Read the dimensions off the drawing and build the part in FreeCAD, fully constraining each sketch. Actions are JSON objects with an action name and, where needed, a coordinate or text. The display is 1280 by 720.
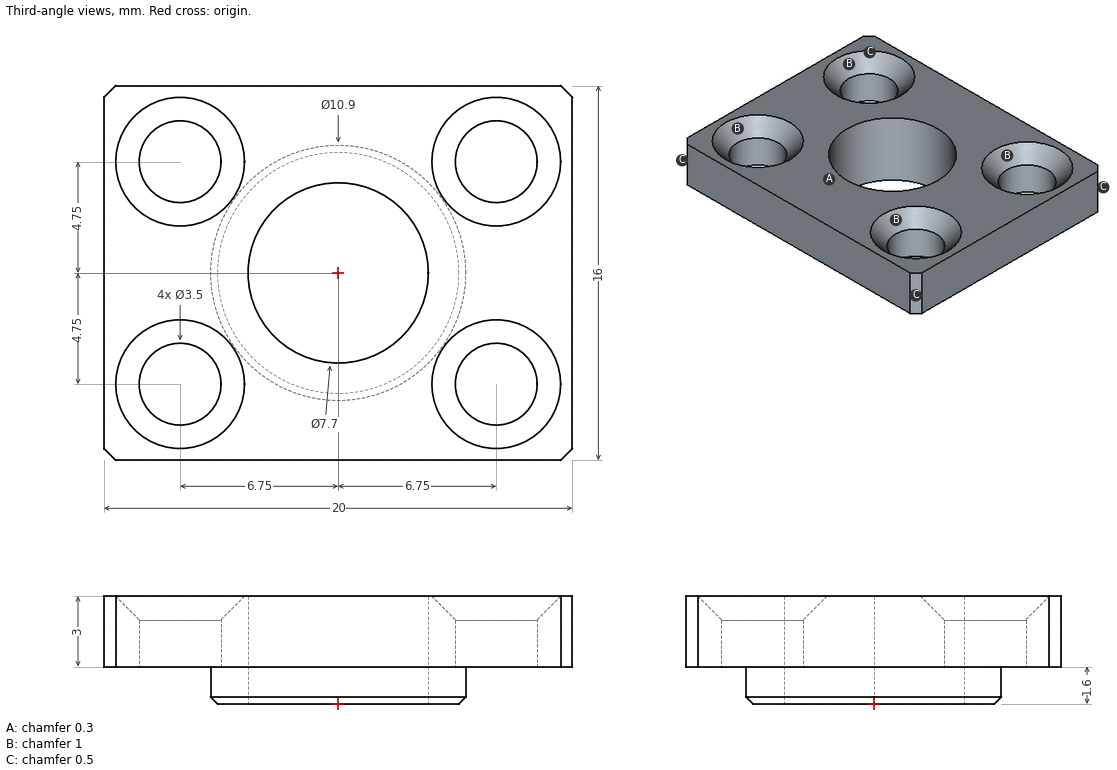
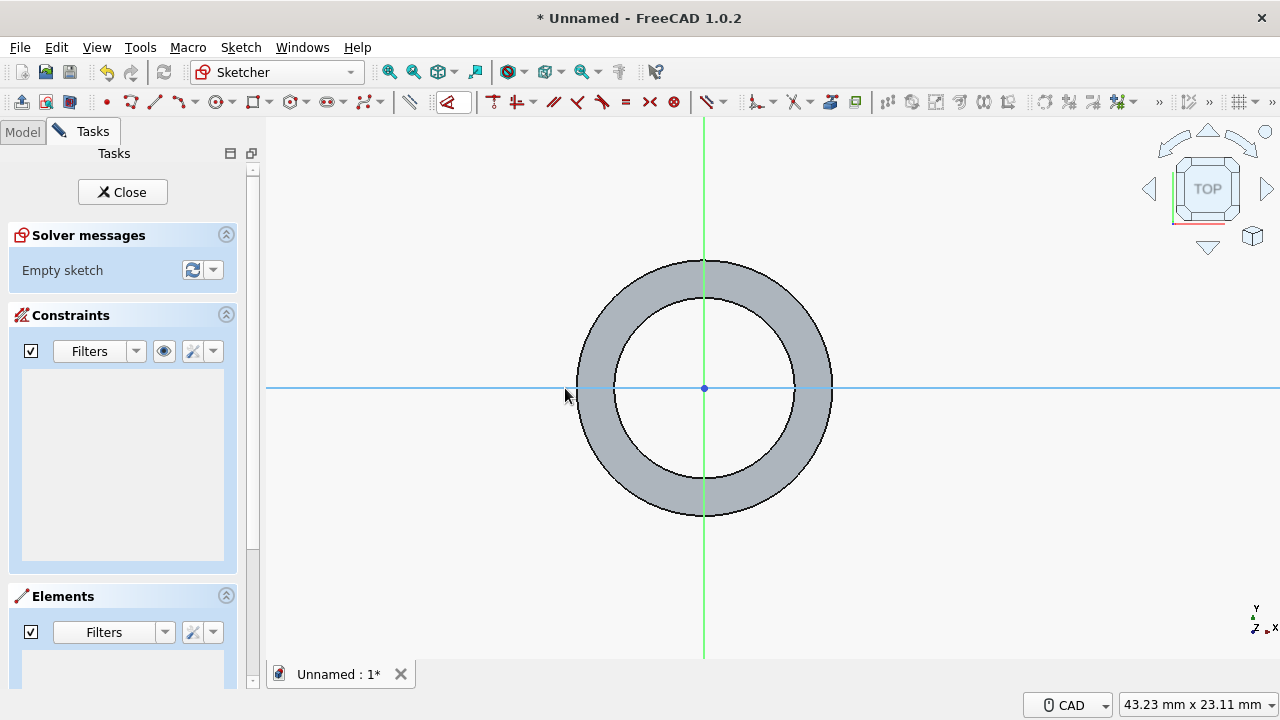
{"action": "key", "text": "g v"}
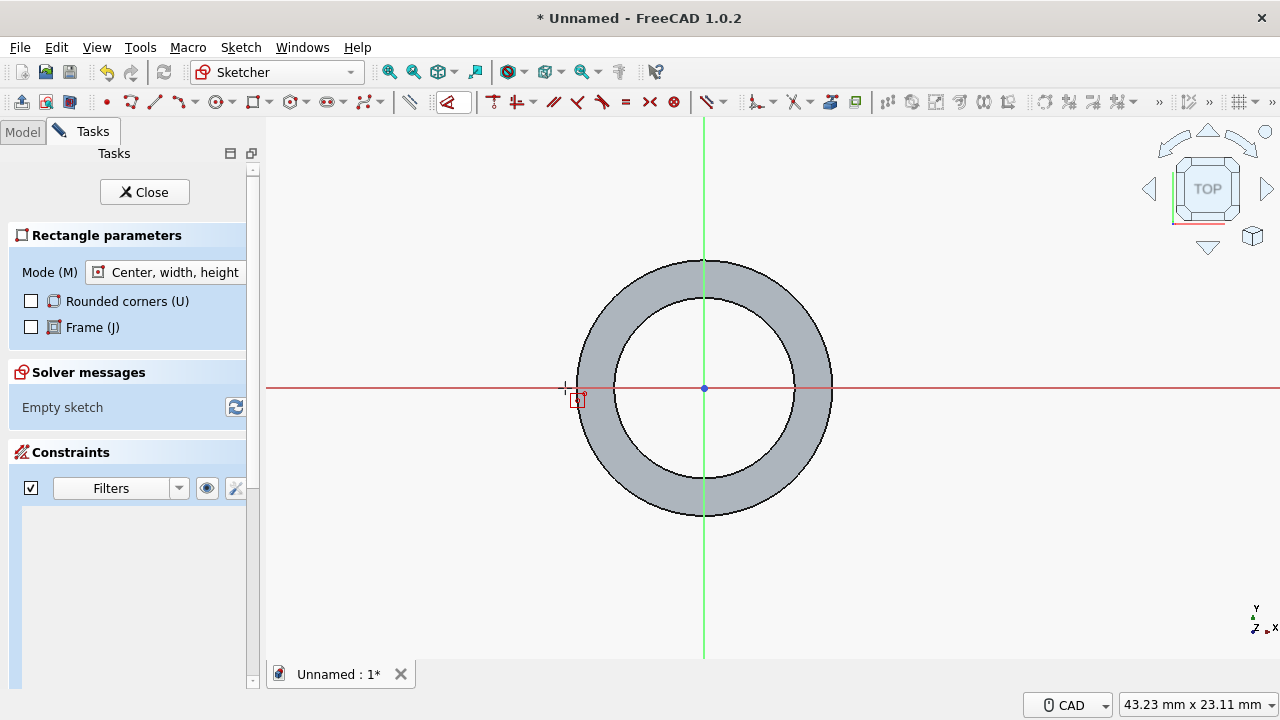
{"action": "left_click", "coordinate": [704, 388]}
{"action": "left_click", "coordinate": [939, 201]}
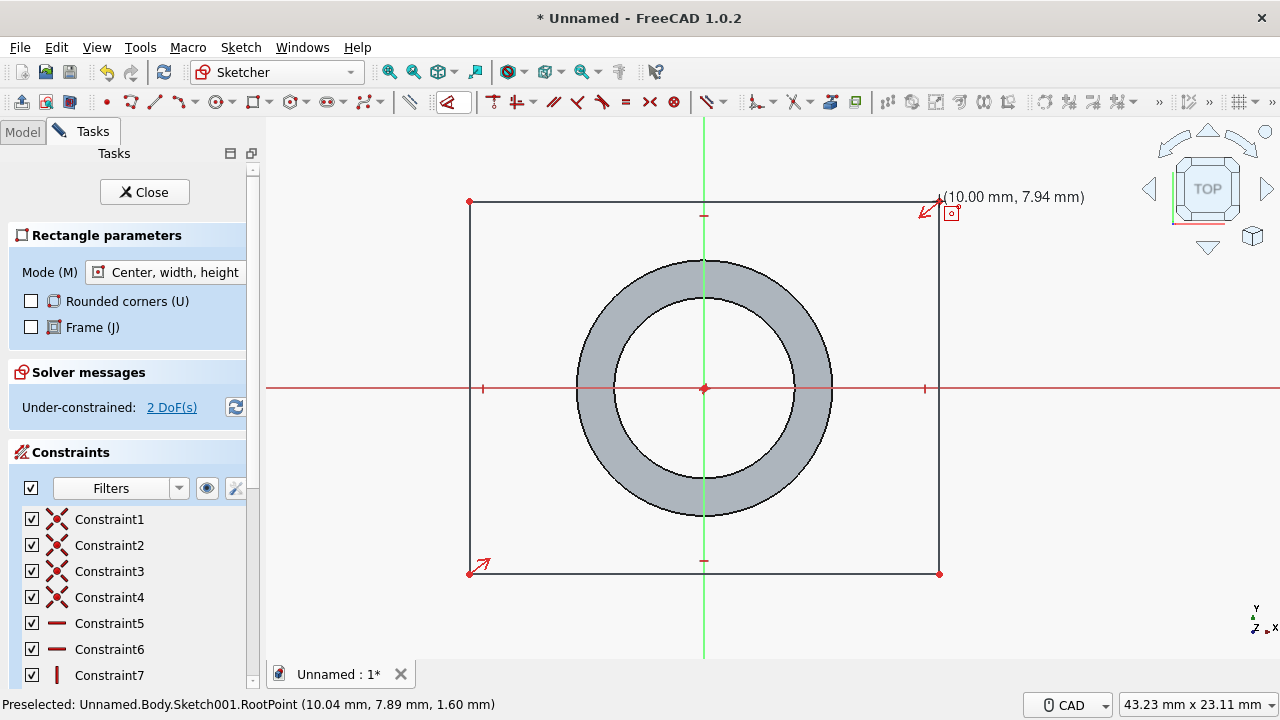
{"action": "key", "text": "g c"}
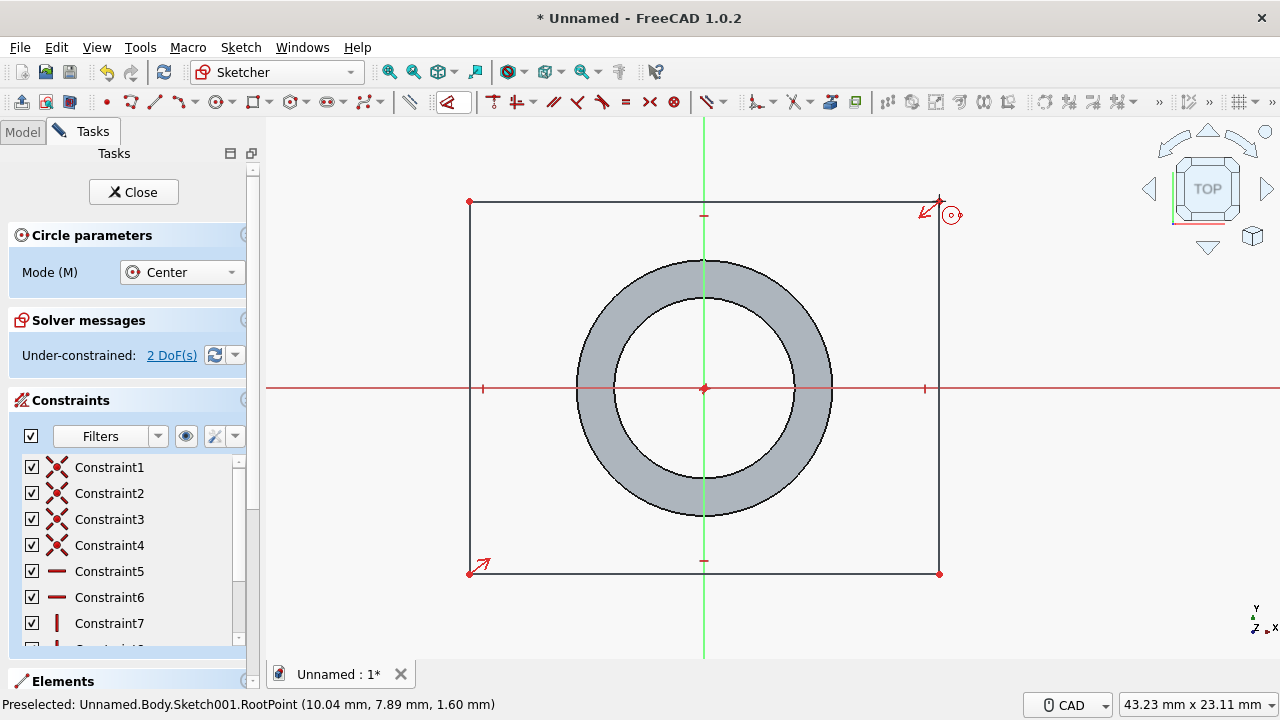
{"action": "left_click", "coordinate": [546, 500]}
{"action": "left_click", "coordinate": [575, 471]}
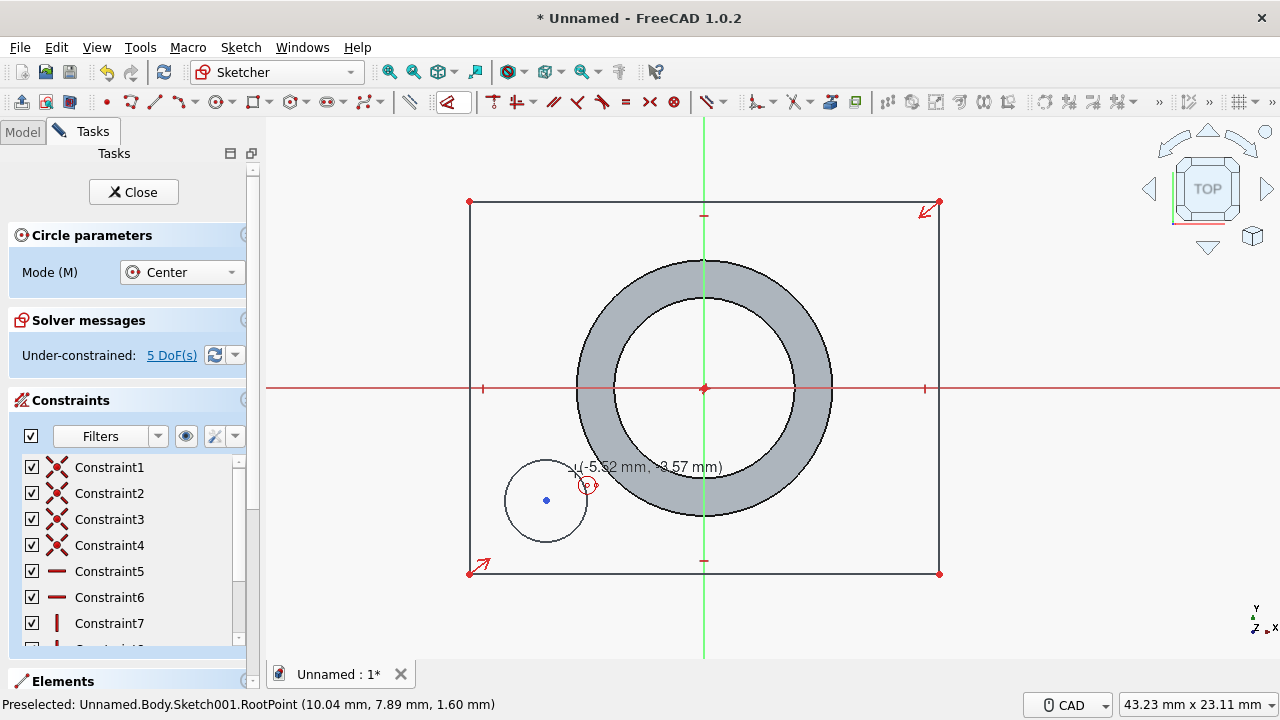
{"action": "left_click", "coordinate": [863, 500]}
{"action": "left_click", "coordinate": [892, 471]}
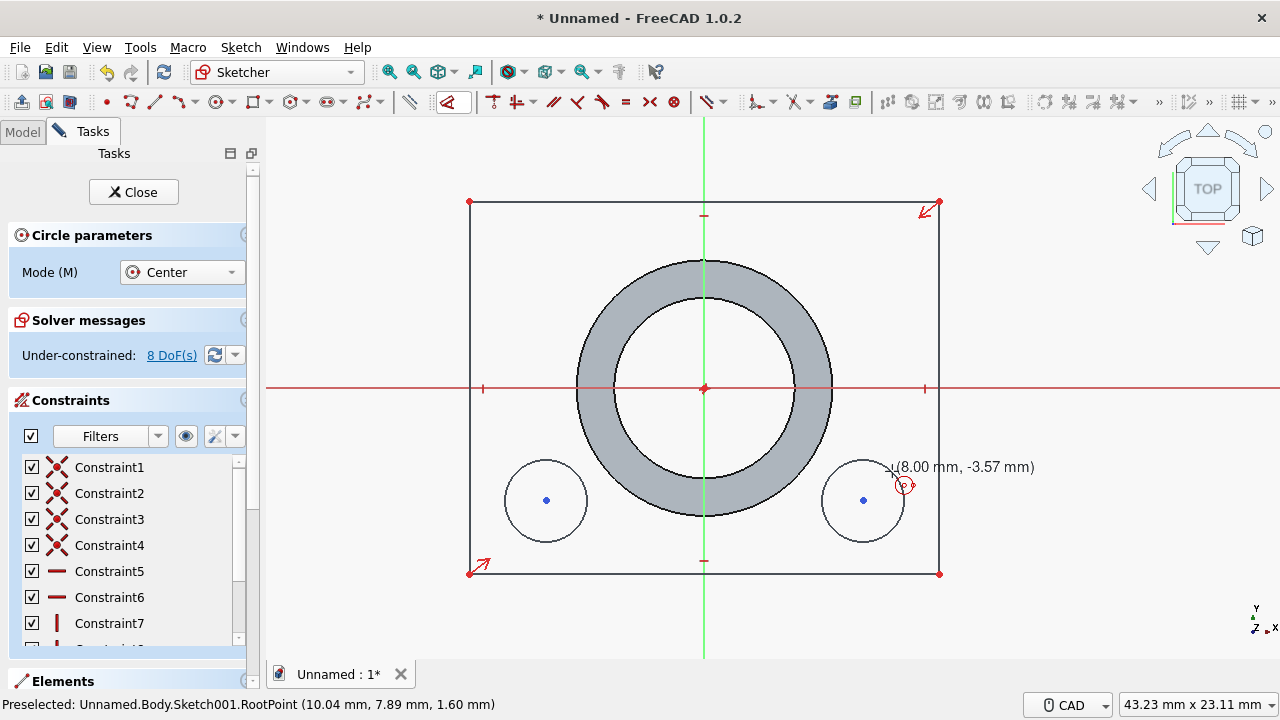
{"action": "left_click", "coordinate": [546, 277]}
{"action": "left_click", "coordinate": [575, 248]}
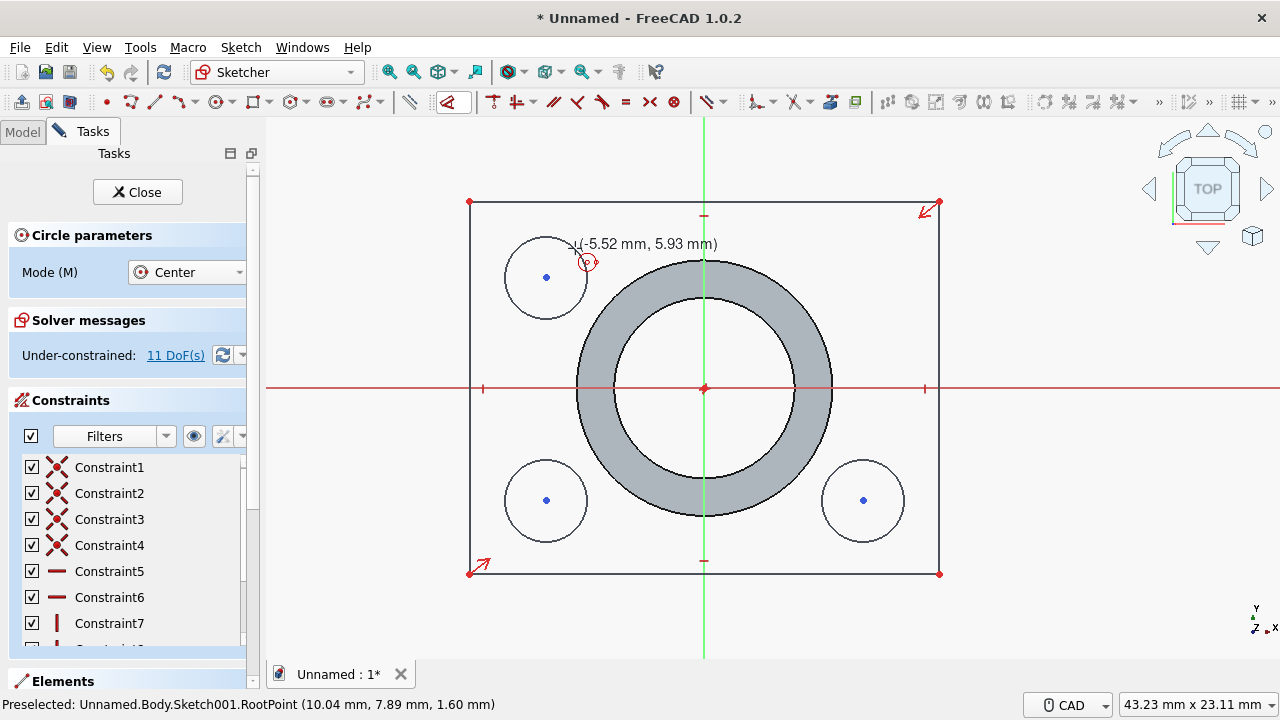
{"action": "left_click", "coordinate": [704, 388]}
{"action": "left_click", "coordinate": [768, 324]}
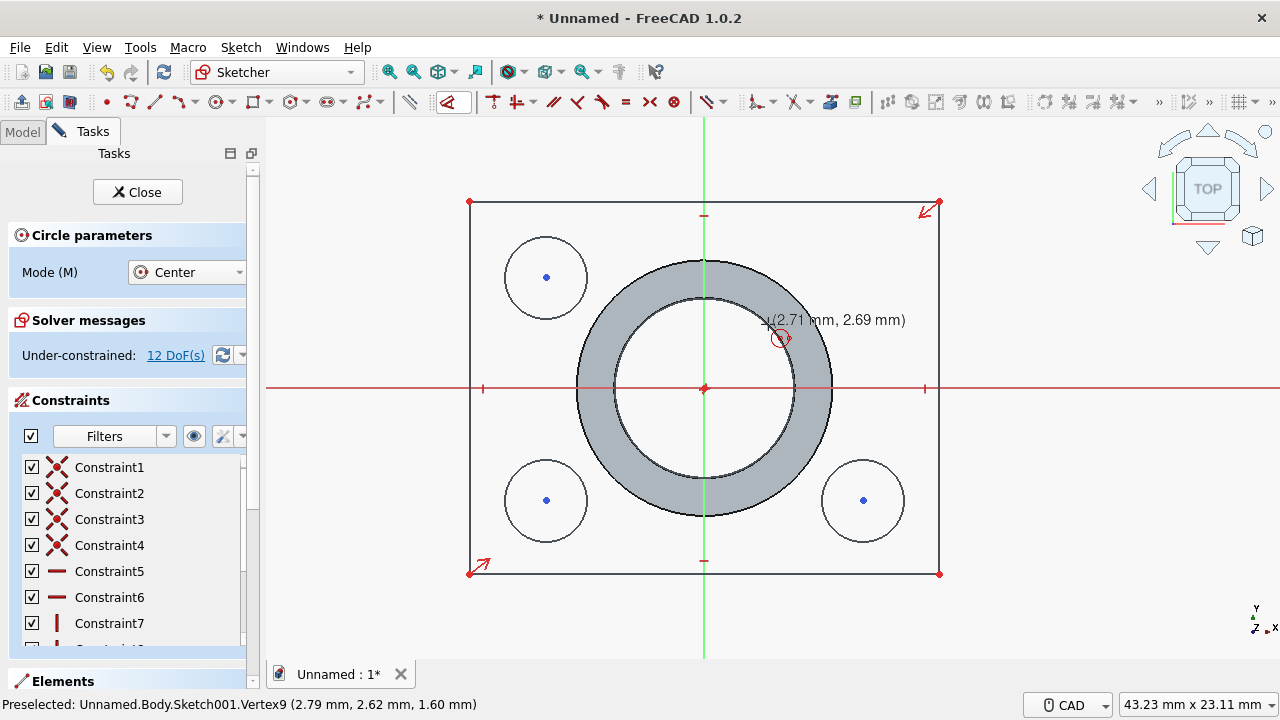
{"action": "left_click", "coordinate": [863, 277]}
{"action": "left_click", "coordinate": [892, 248]}
{"action": "key", "text": "Escape"}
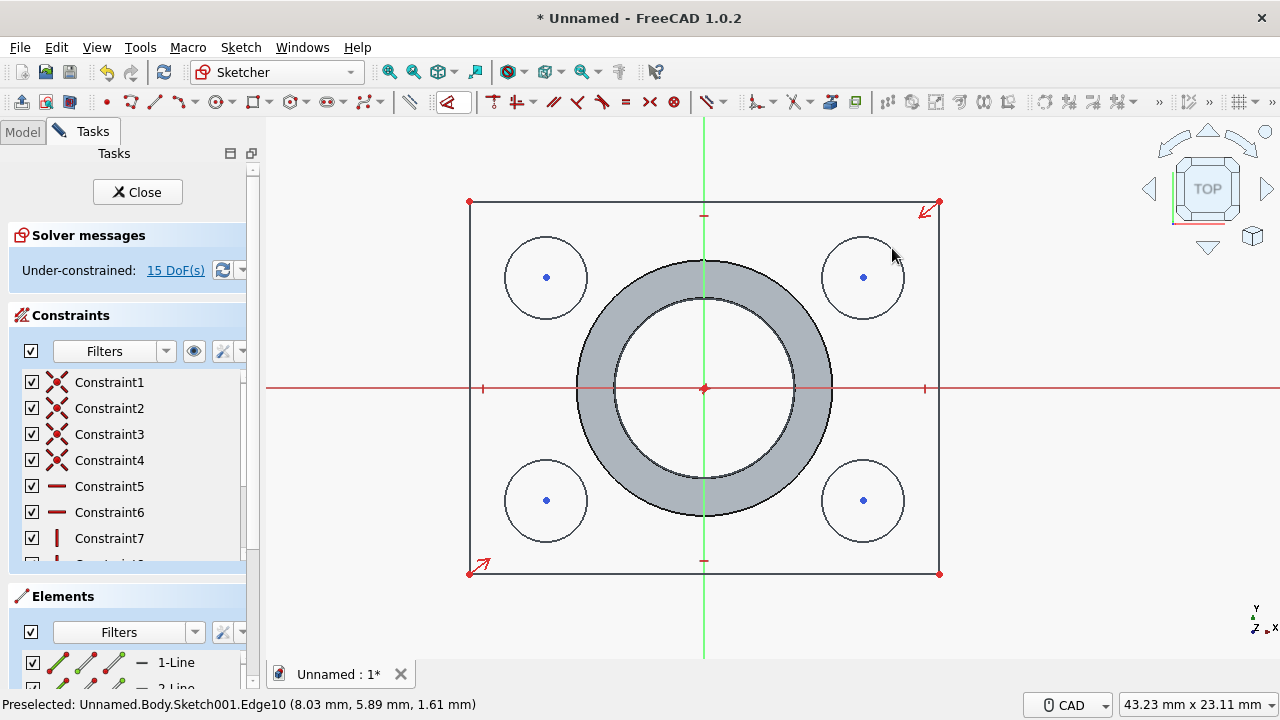
{"action": "left_click", "coordinate": [575, 472]}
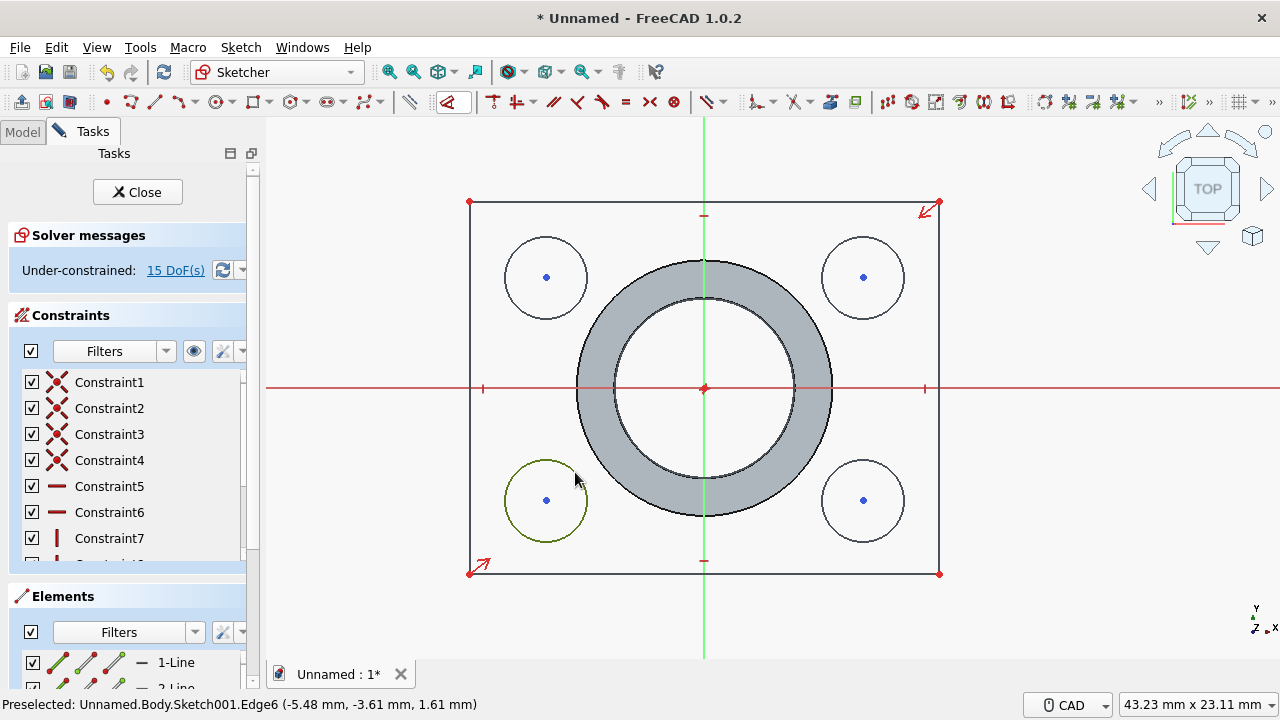
{"action": "left_click", "coordinate": [892, 472]}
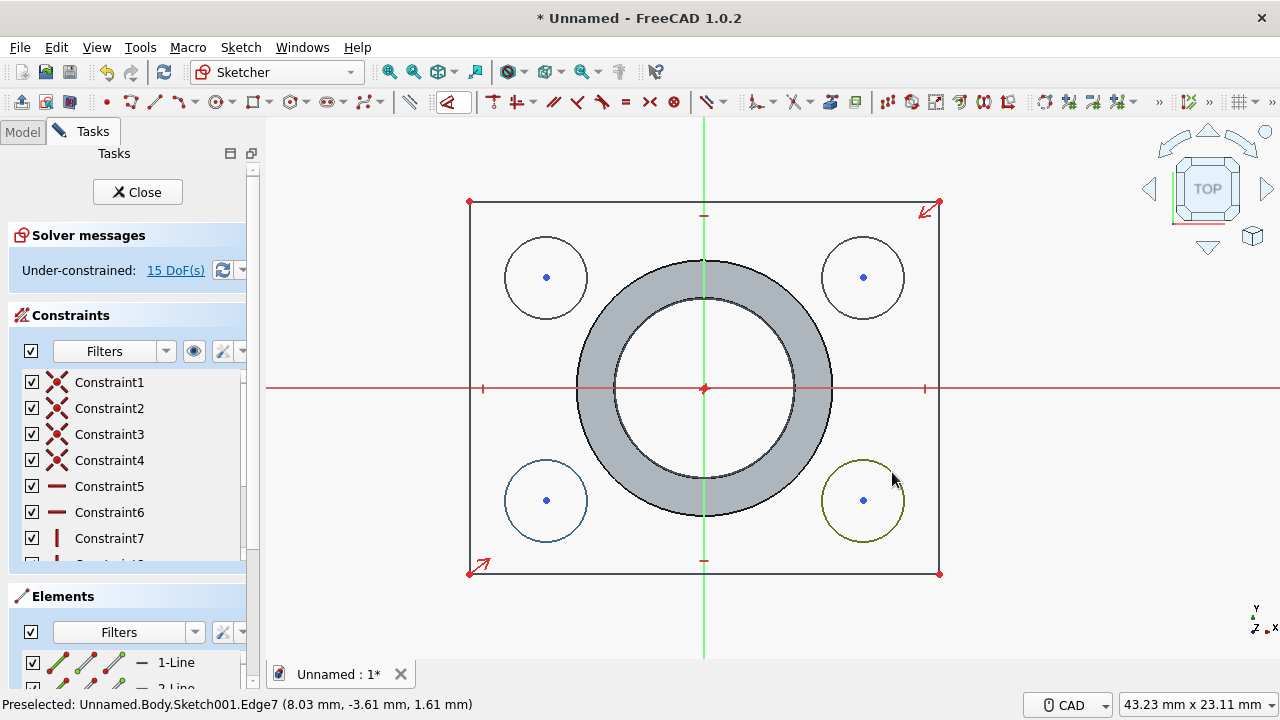
{"action": "left_click", "coordinate": [575, 249]}